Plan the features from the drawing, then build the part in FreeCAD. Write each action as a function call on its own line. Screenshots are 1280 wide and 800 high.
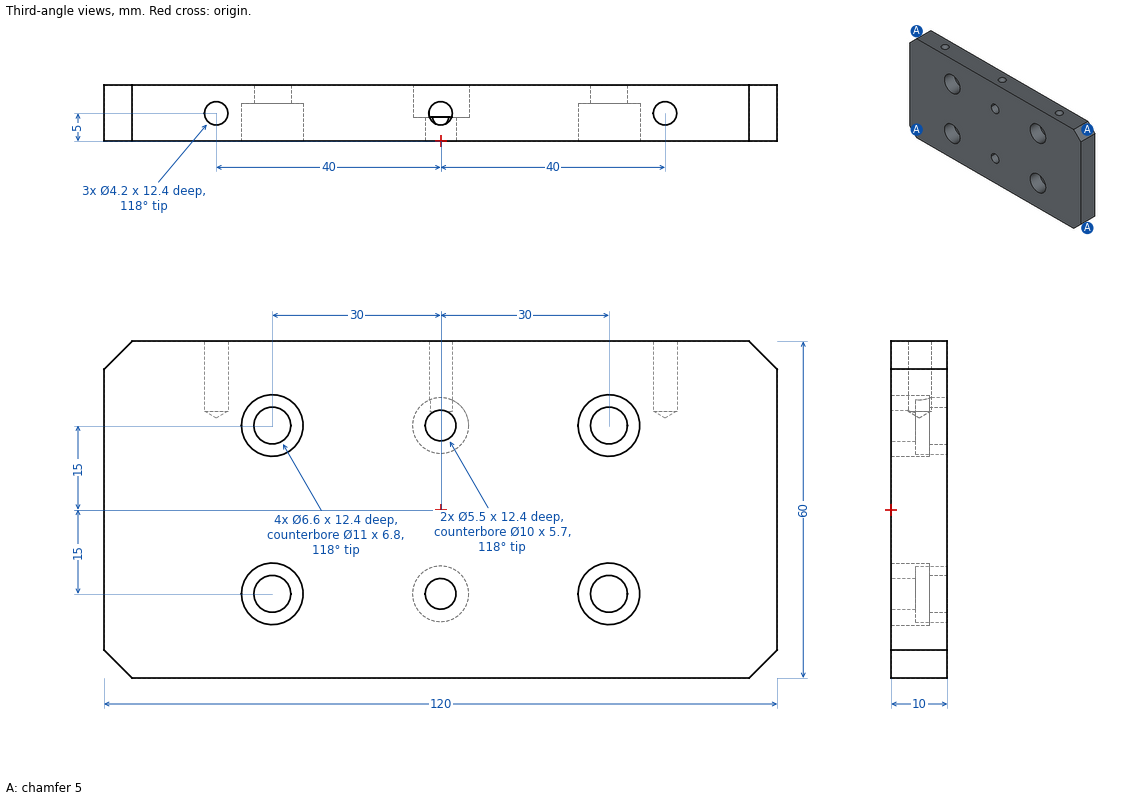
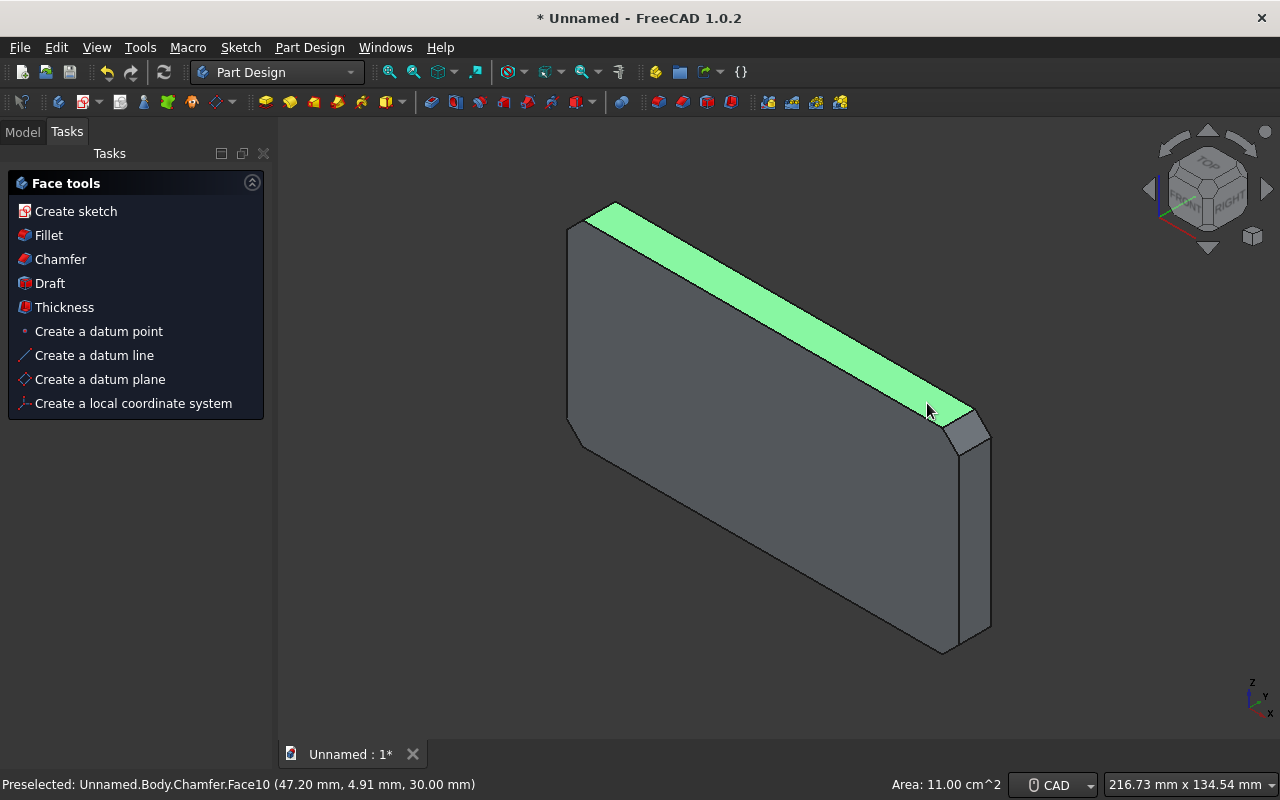
click(84, 102)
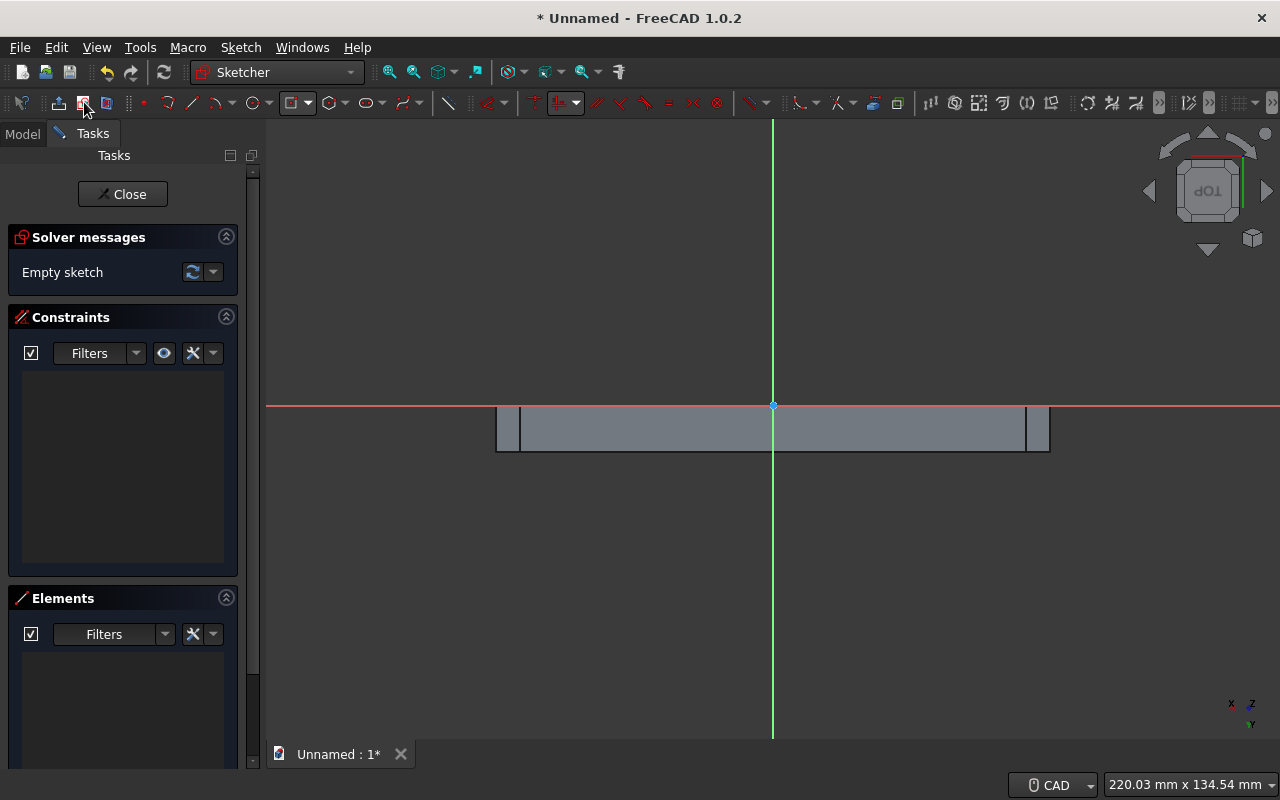
scroll(912, 409, up, 2)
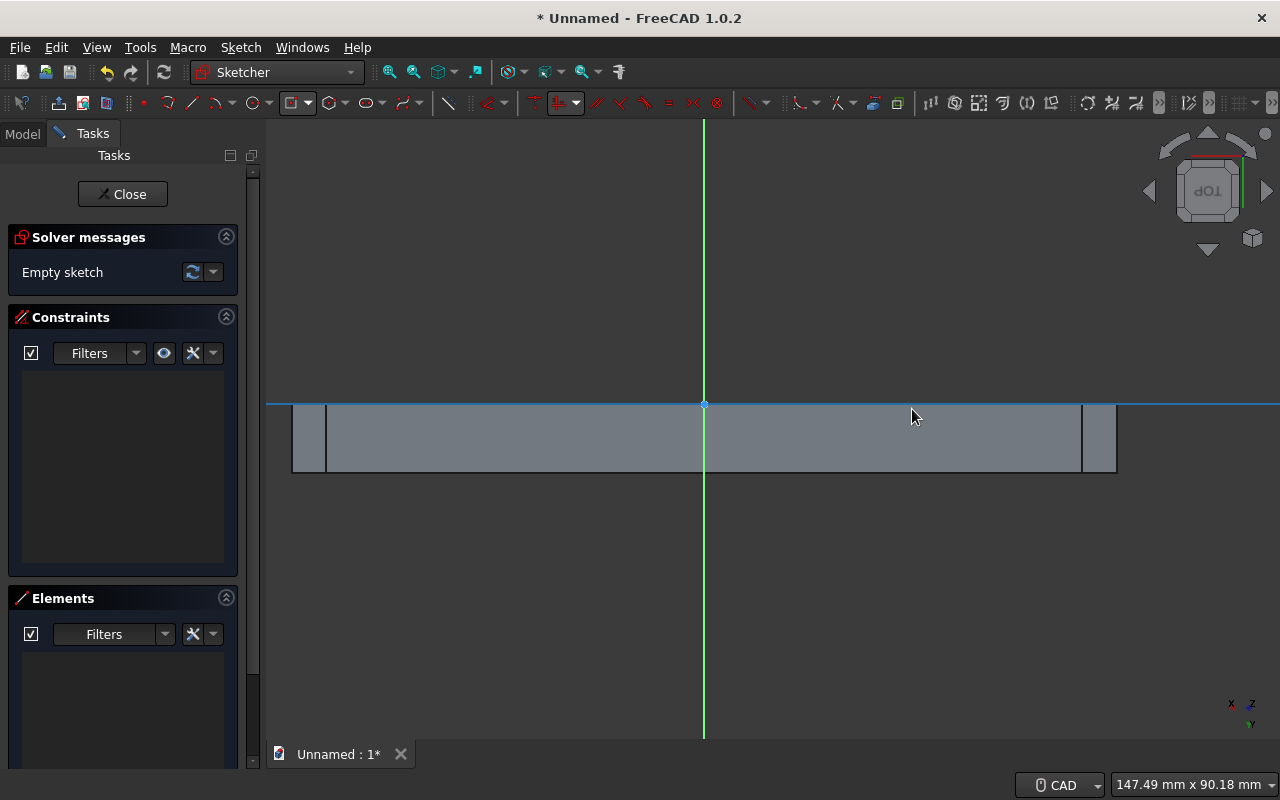
key(g)
key(c)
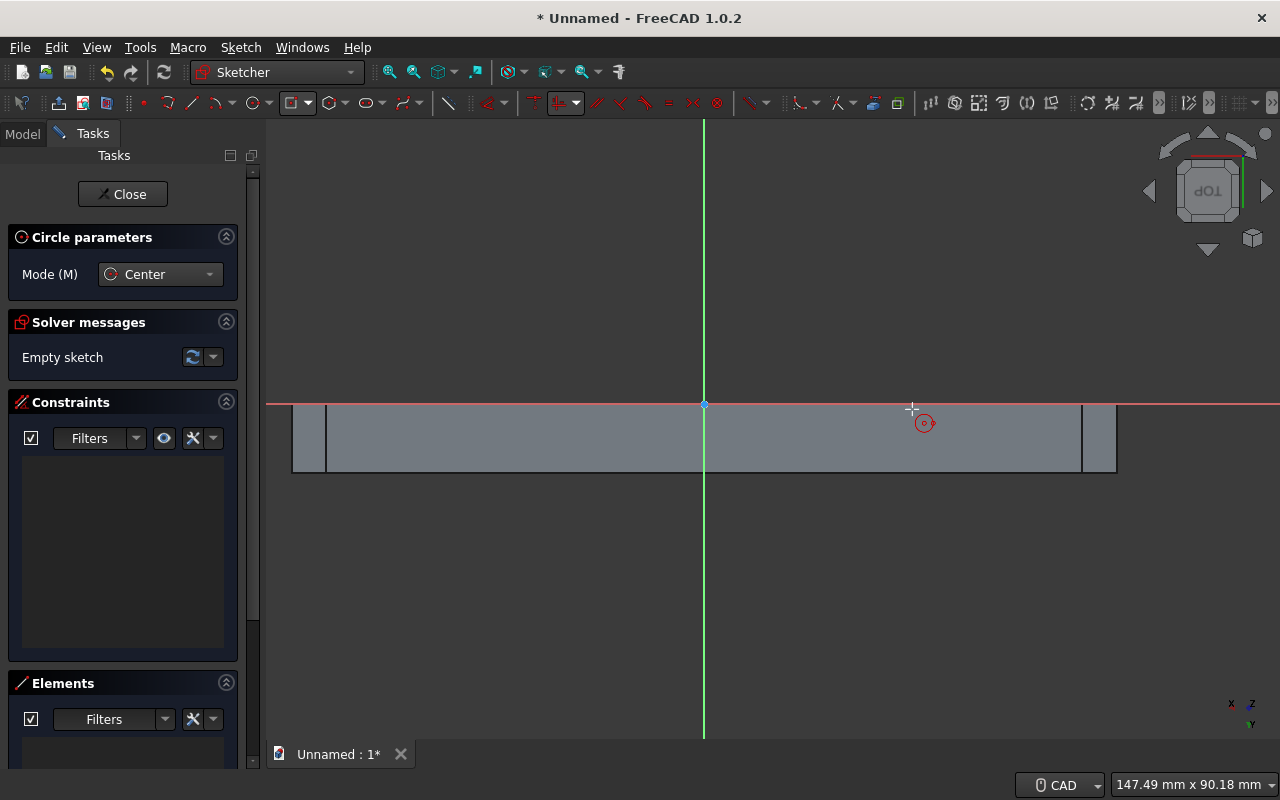
scroll(979, 439, up, 3)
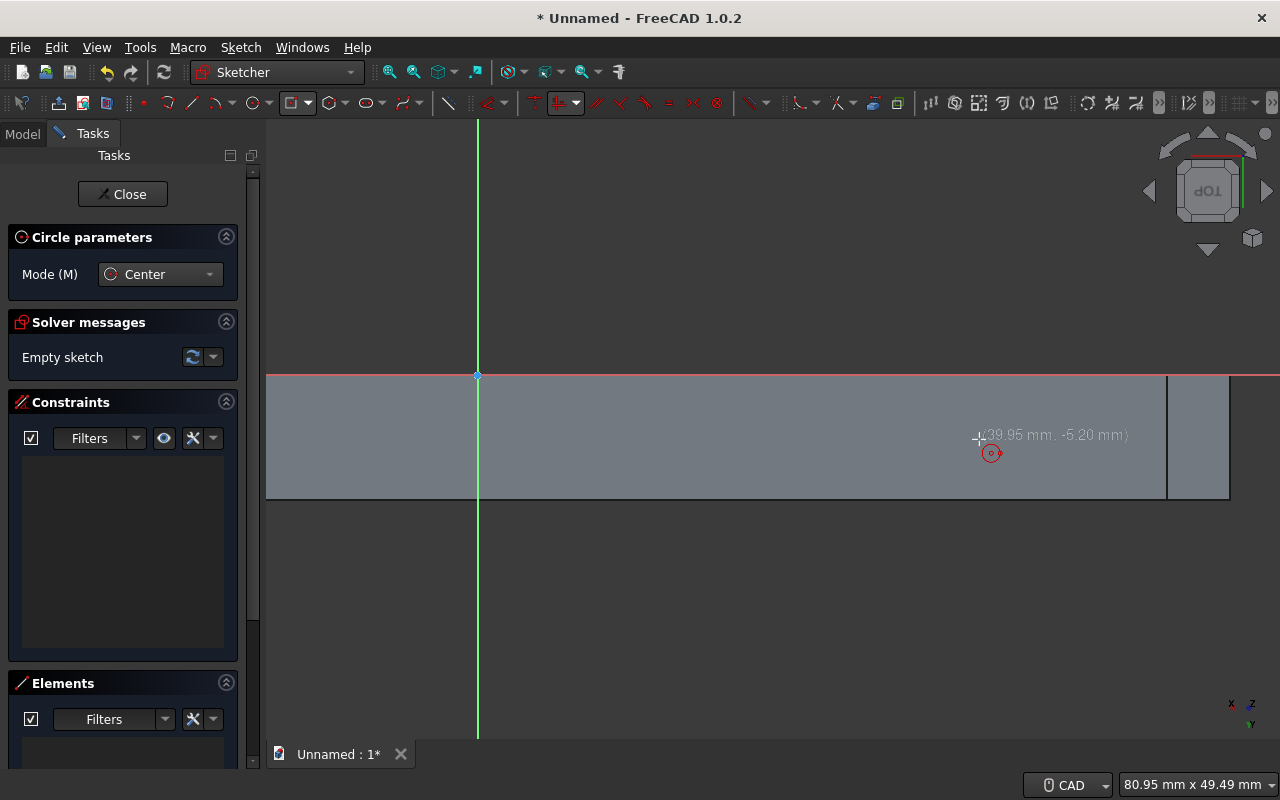
click(979, 438)
move(998, 419)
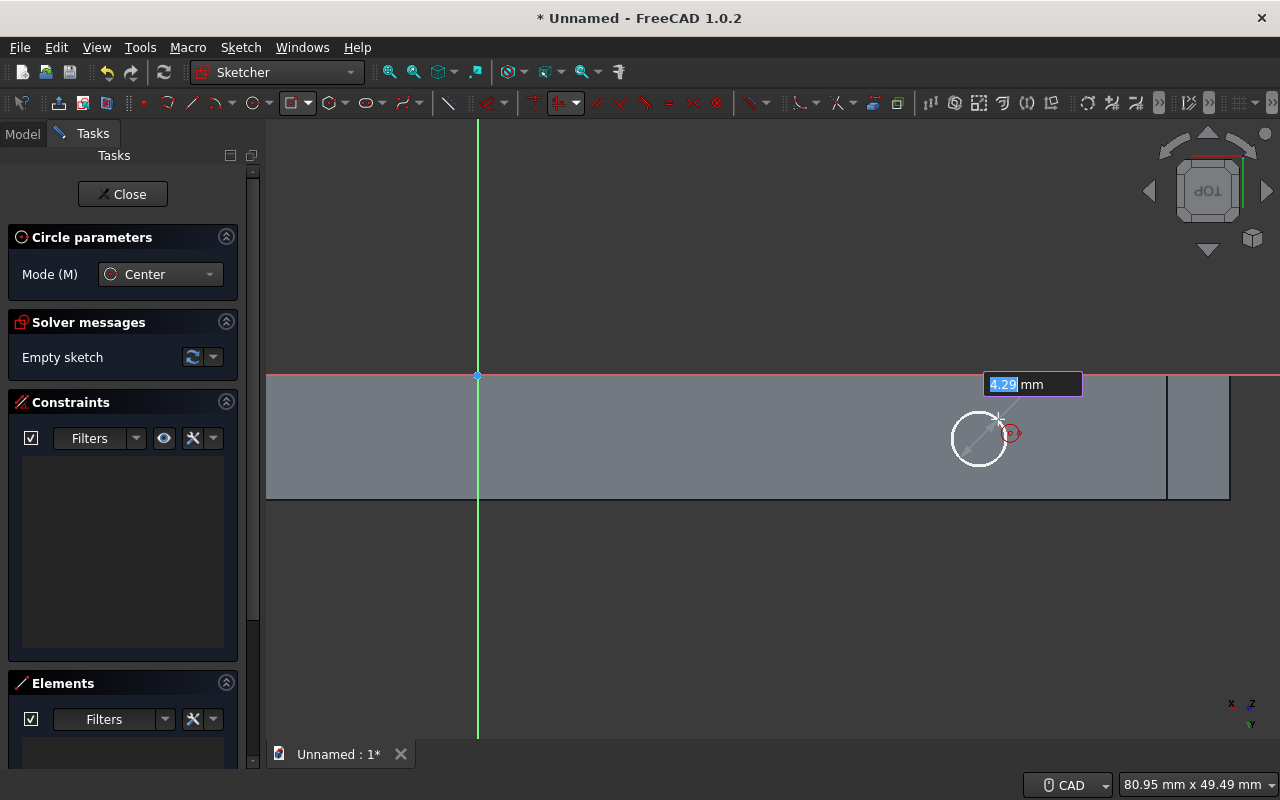
text(4.2)
key(Return)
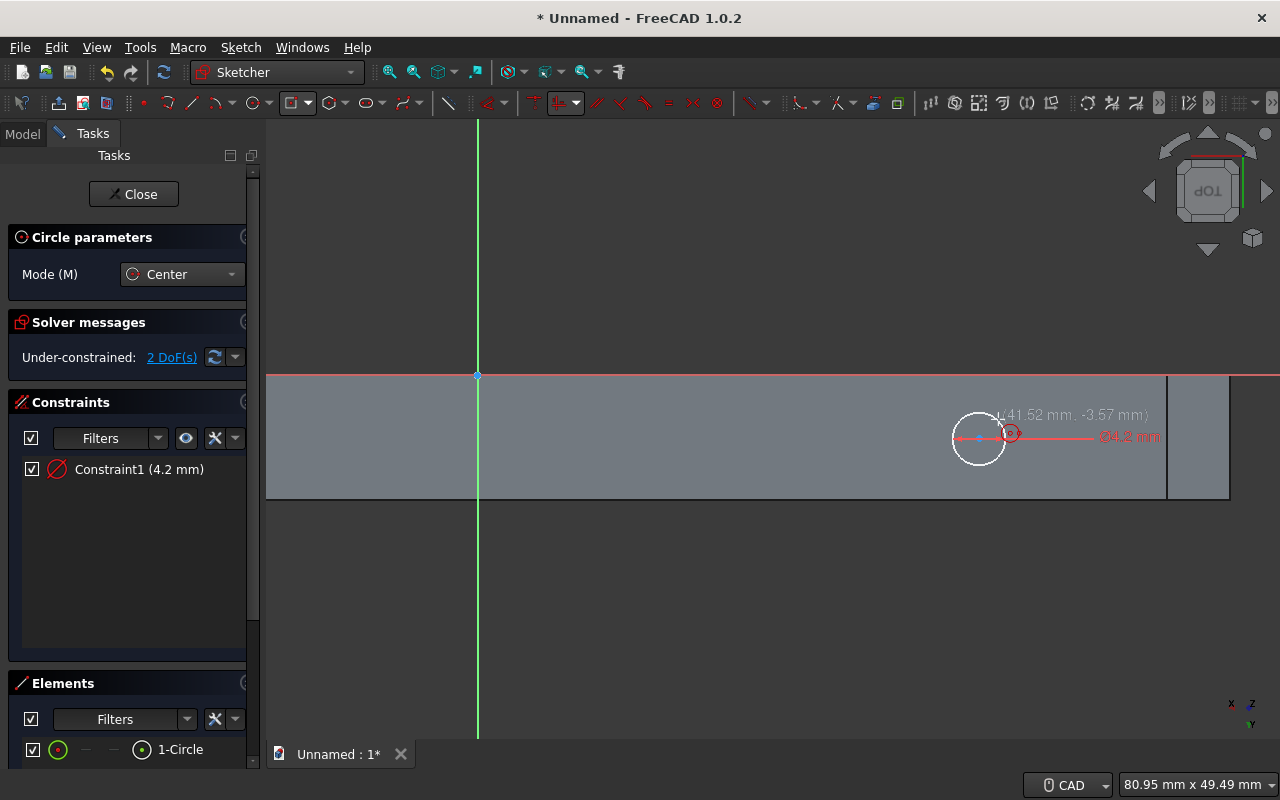
click(478, 438)
move(497, 419)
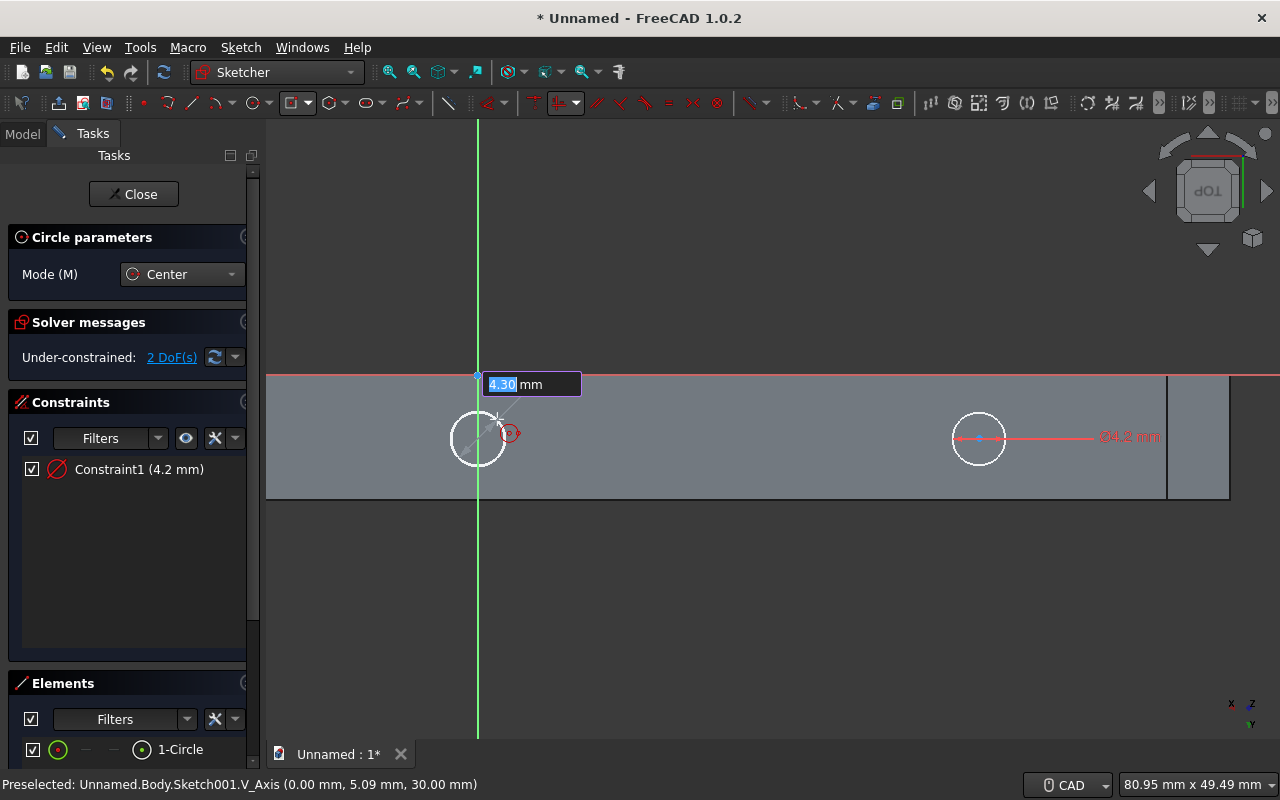
text(4.2)
key(Return)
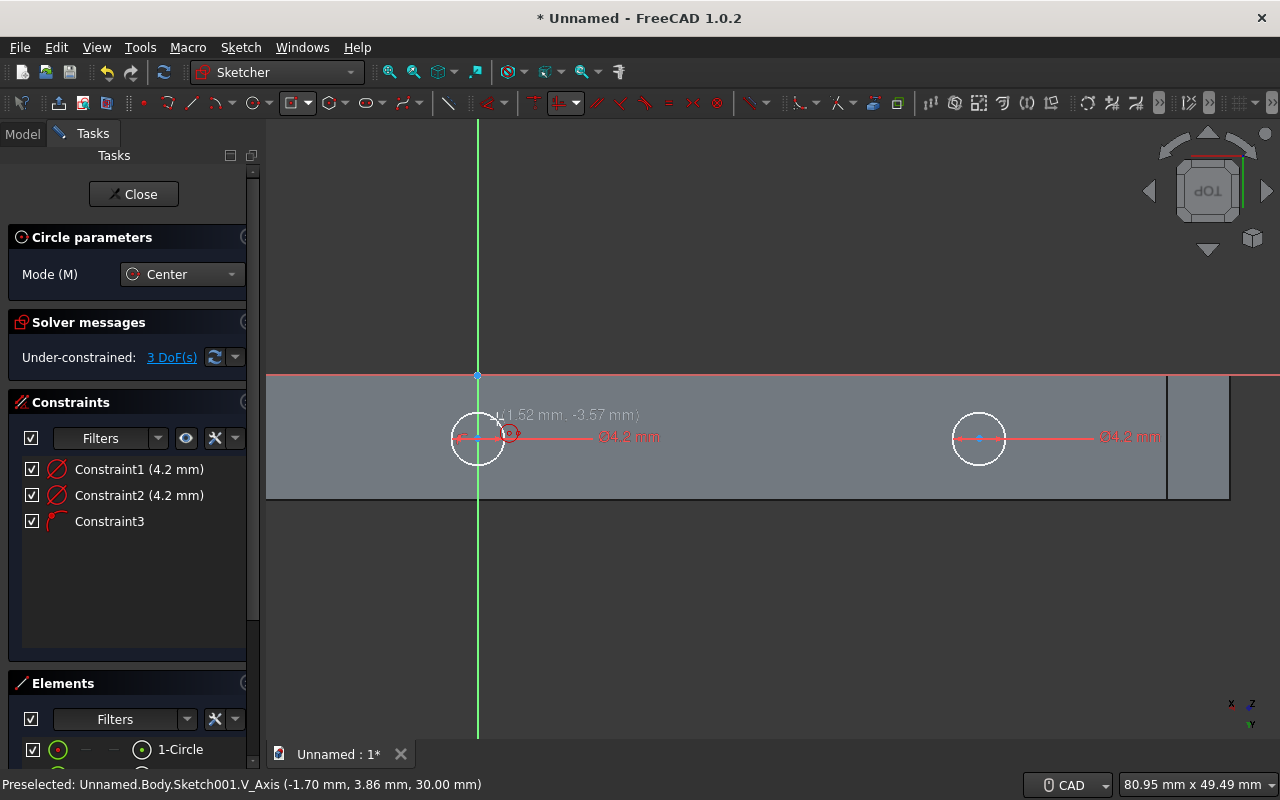
scroll(980, 440, down, 3)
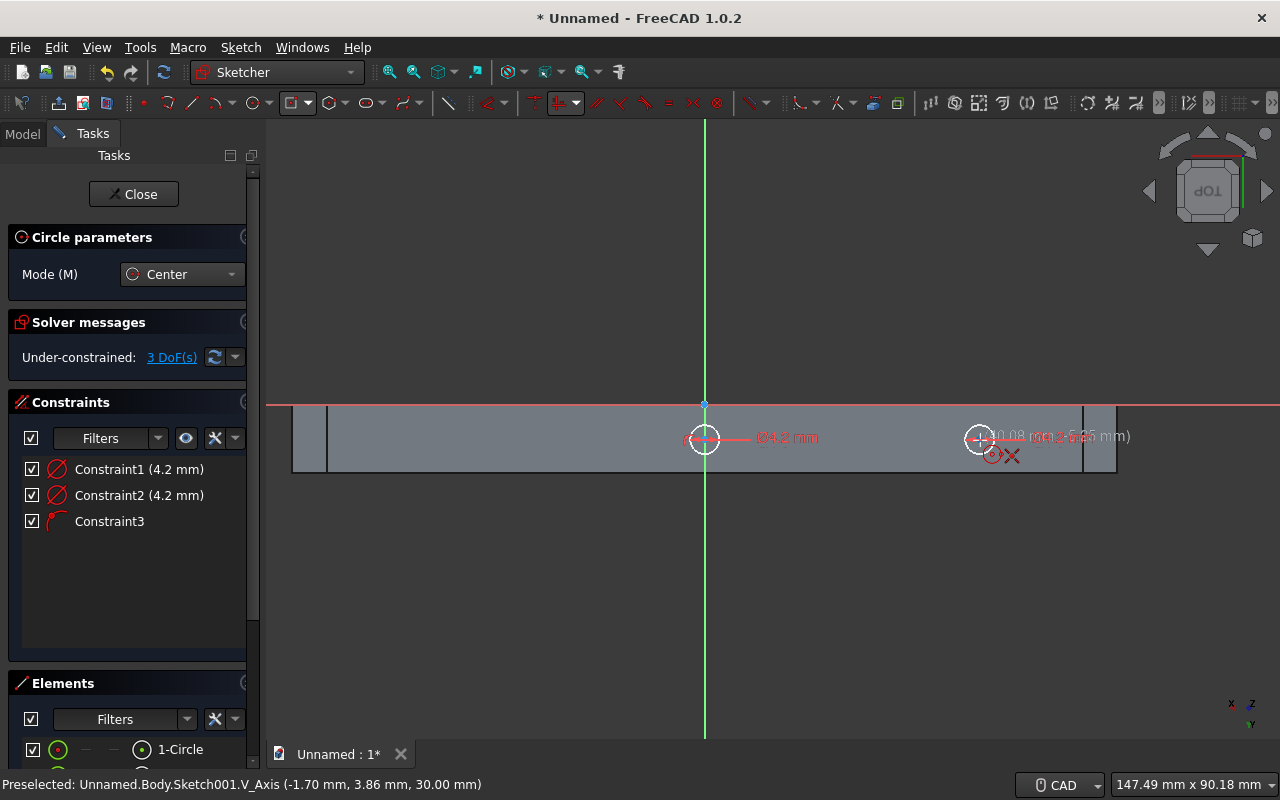
scroll(430, 439, up, 3)